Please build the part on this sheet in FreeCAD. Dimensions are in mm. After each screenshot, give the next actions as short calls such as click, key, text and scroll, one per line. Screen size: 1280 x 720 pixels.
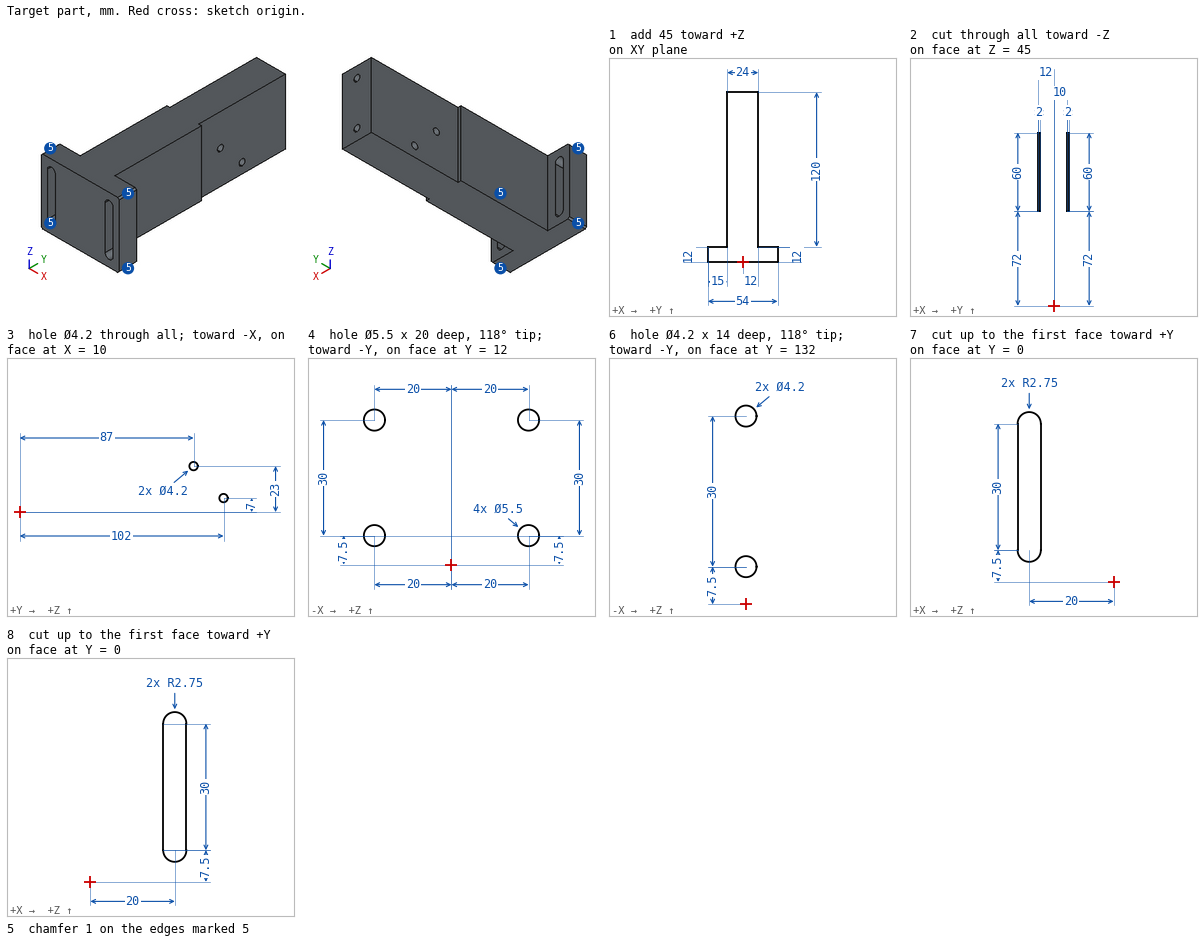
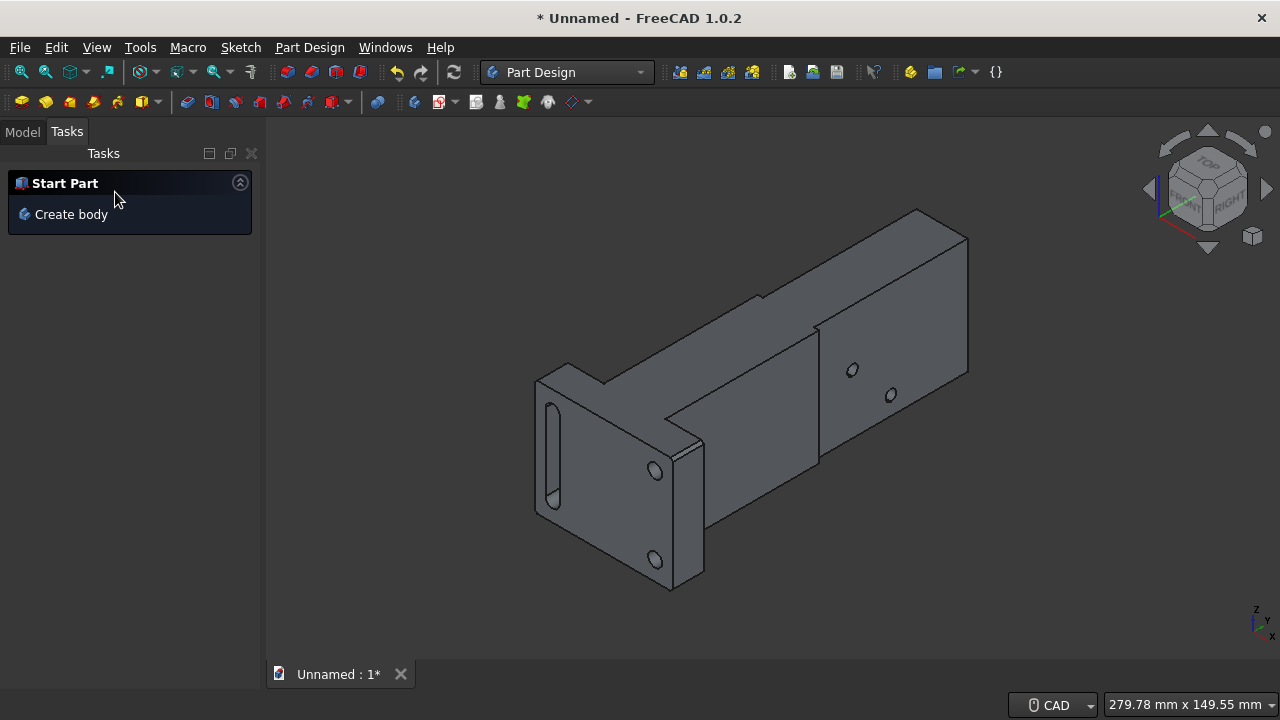
click(604, 485)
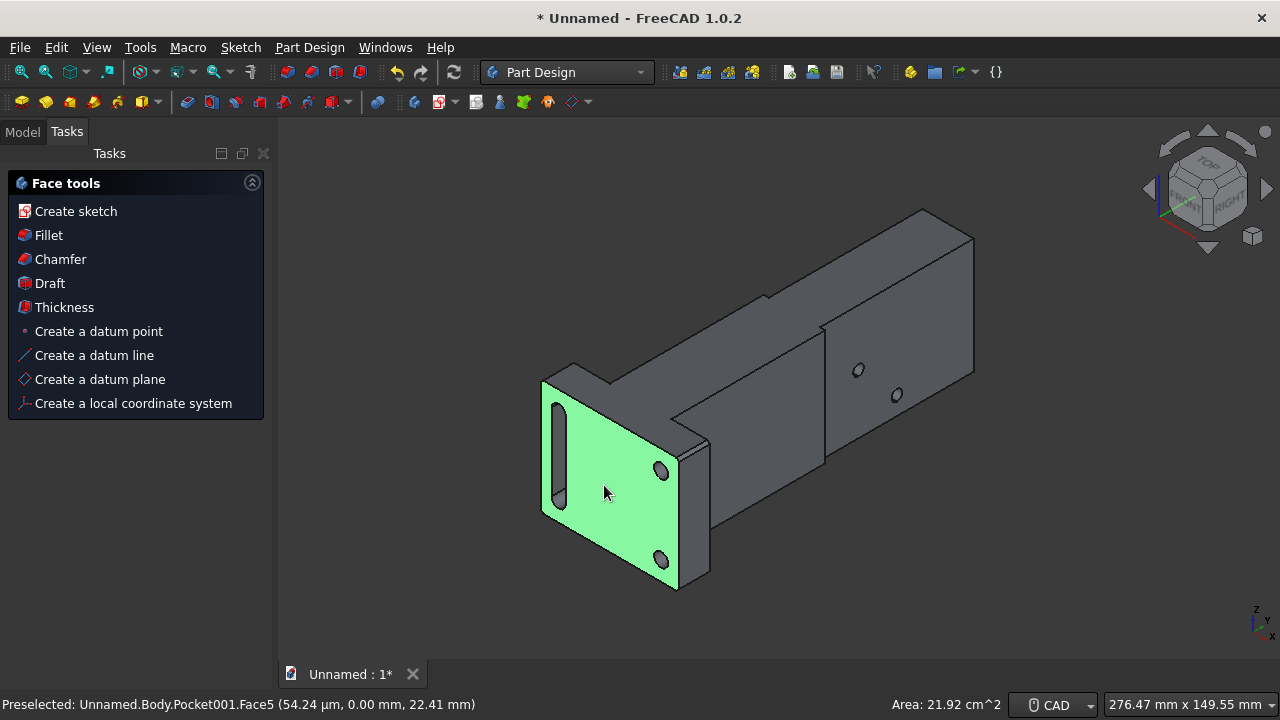
click(440, 102)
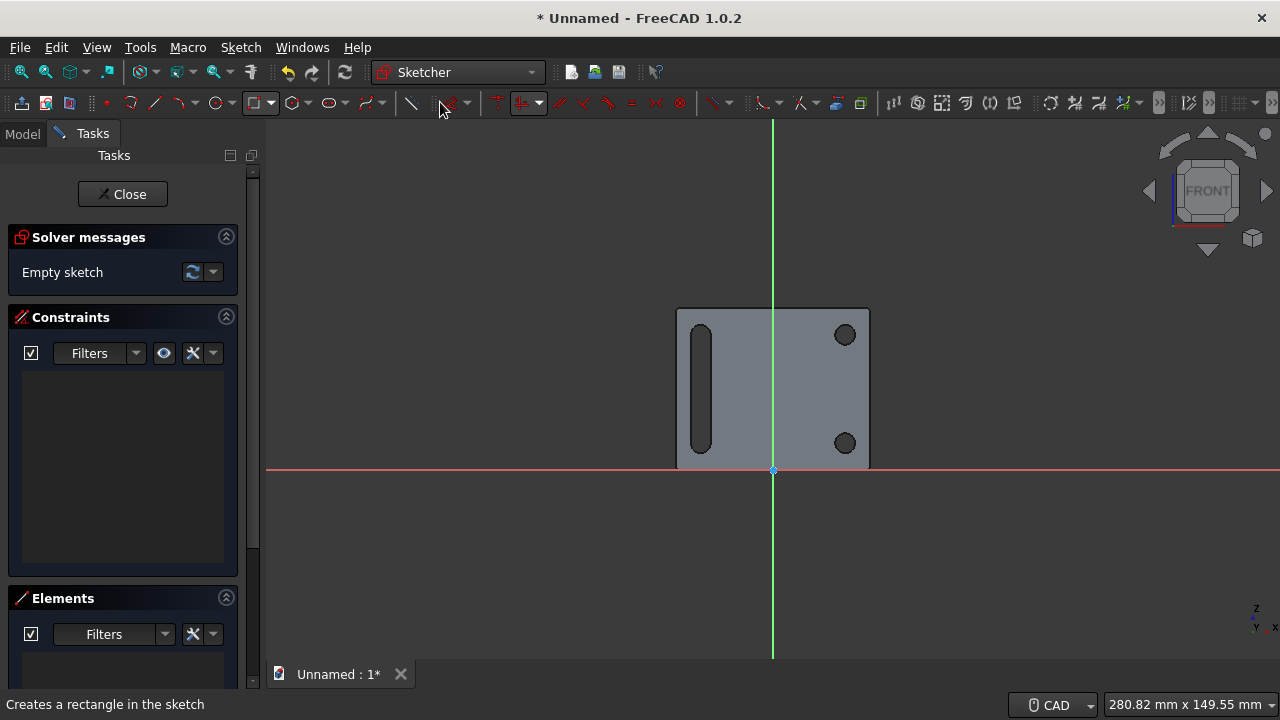
scroll(903, 405, up, 4)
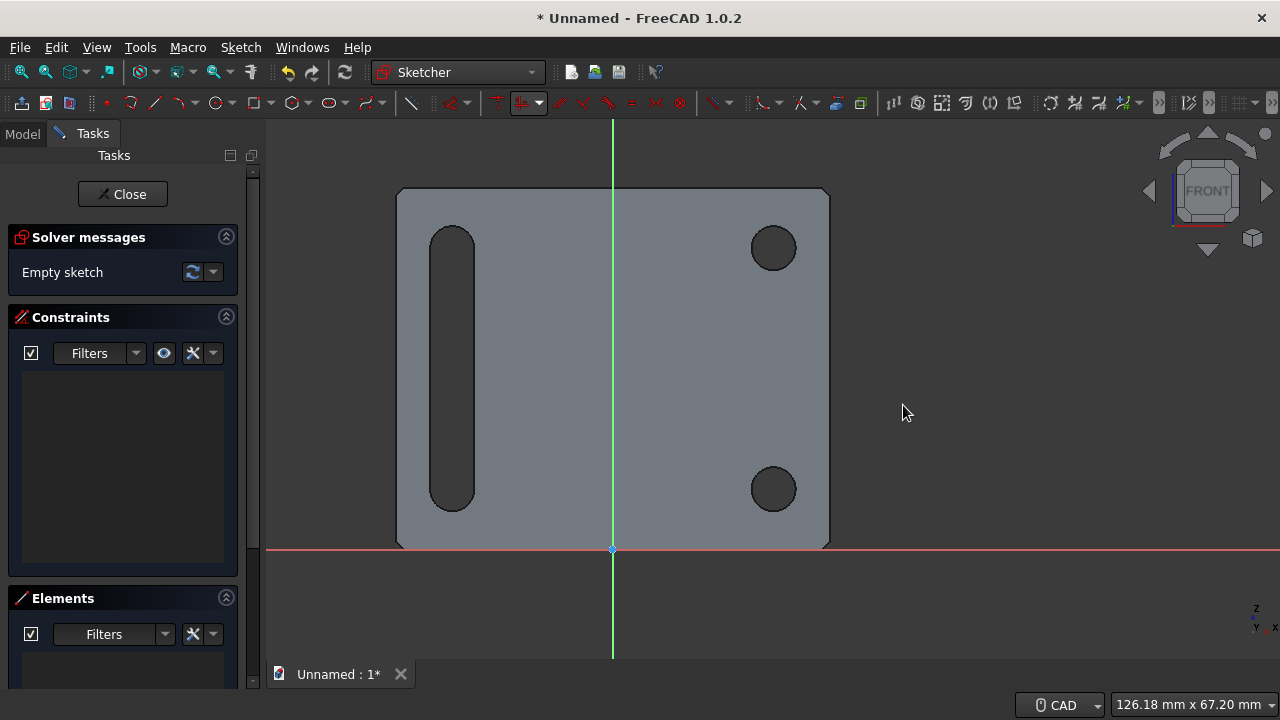
click(330, 104)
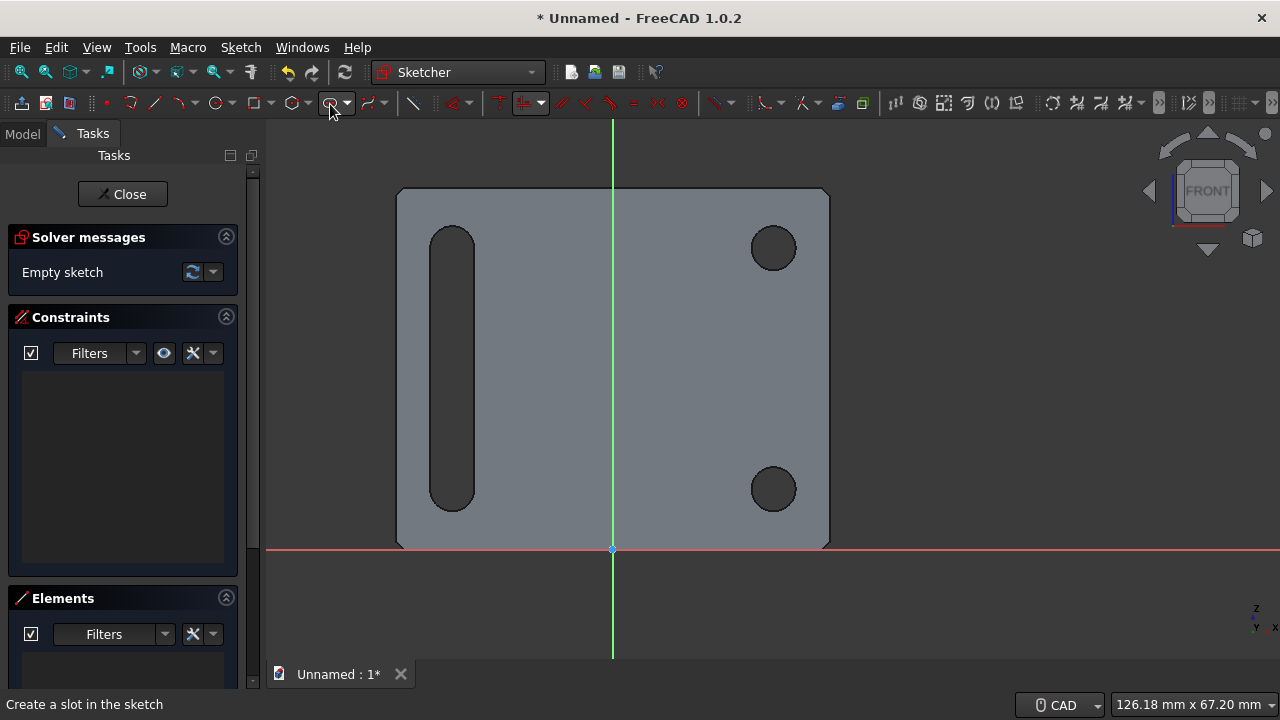
click(774, 489)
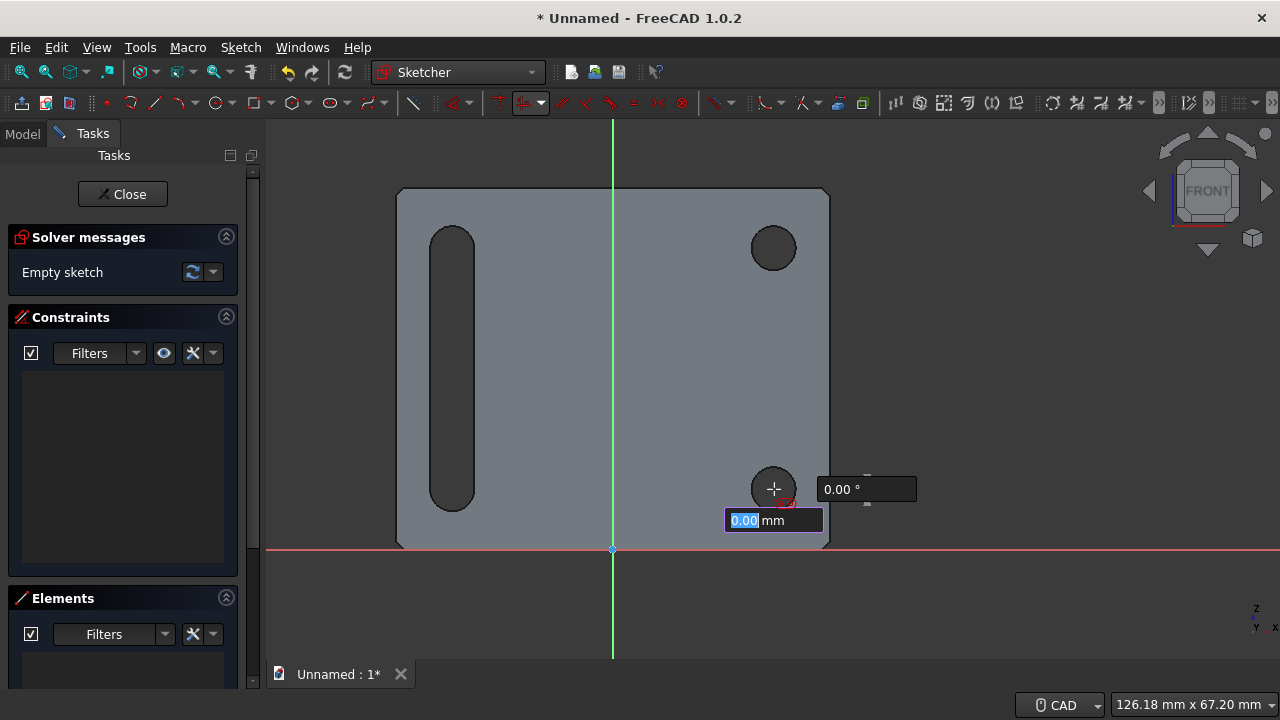
click(774, 248)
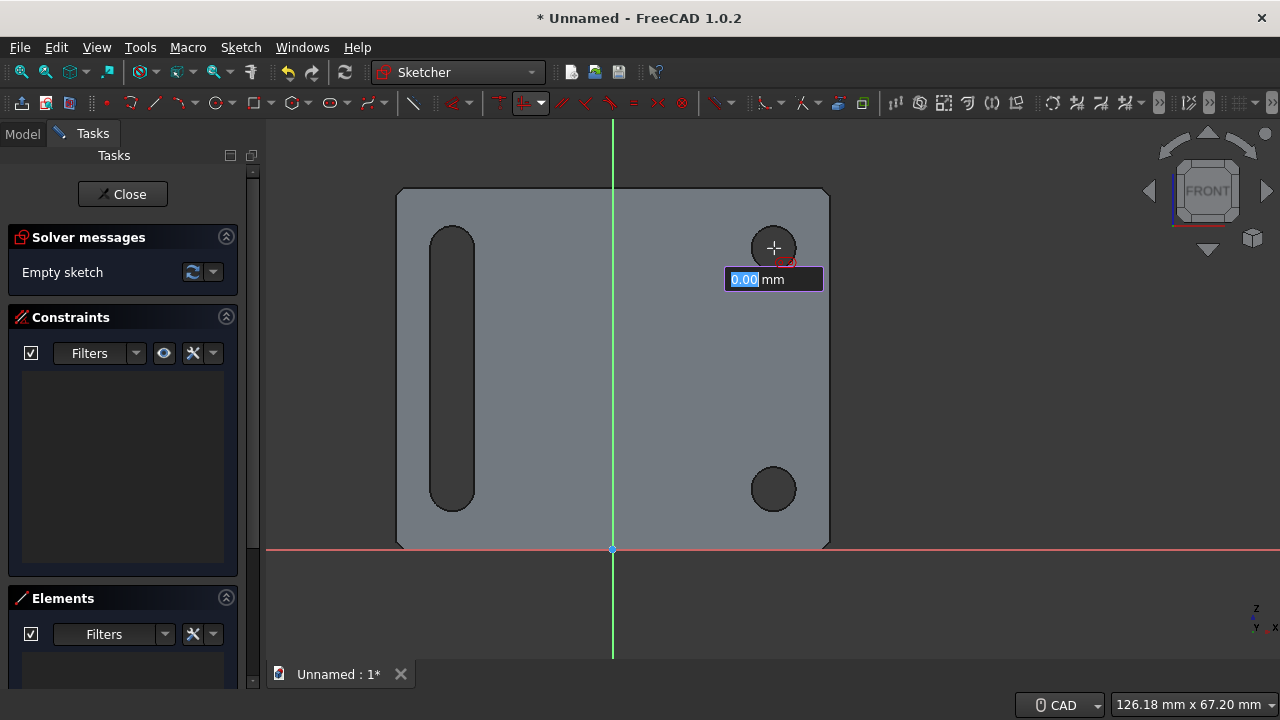
click(796, 369)
key(Escape)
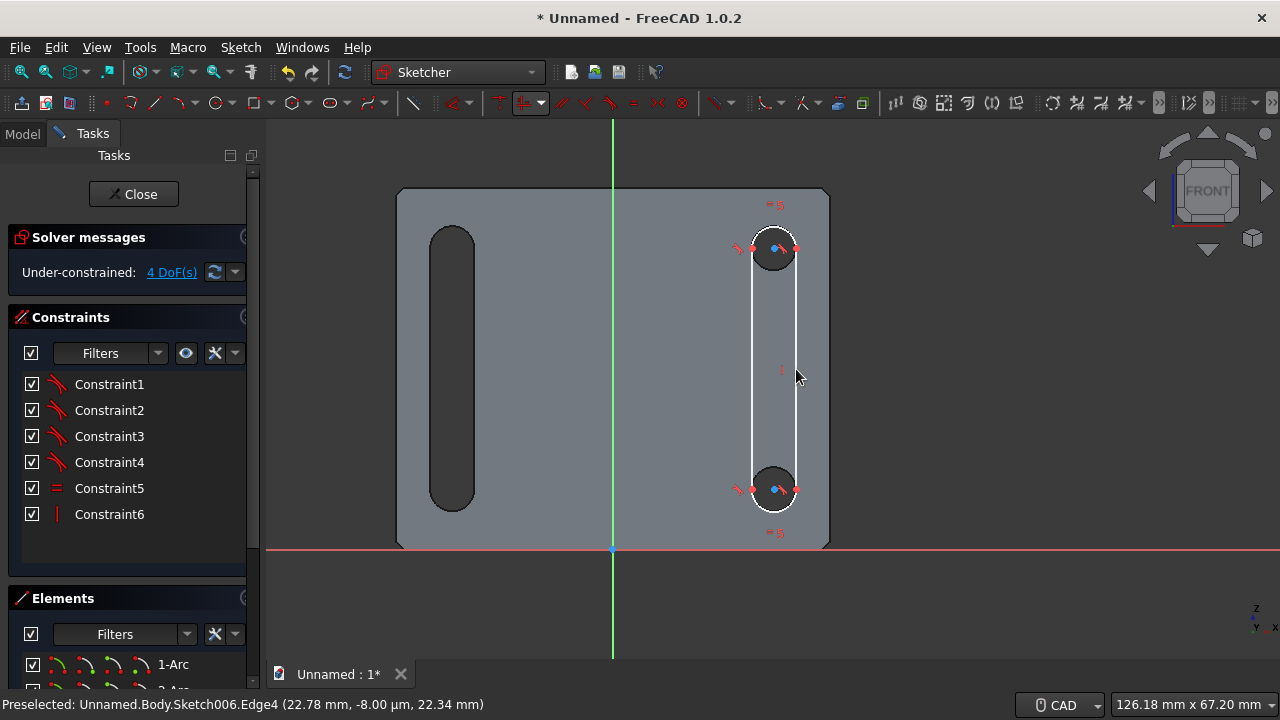
click(452, 104)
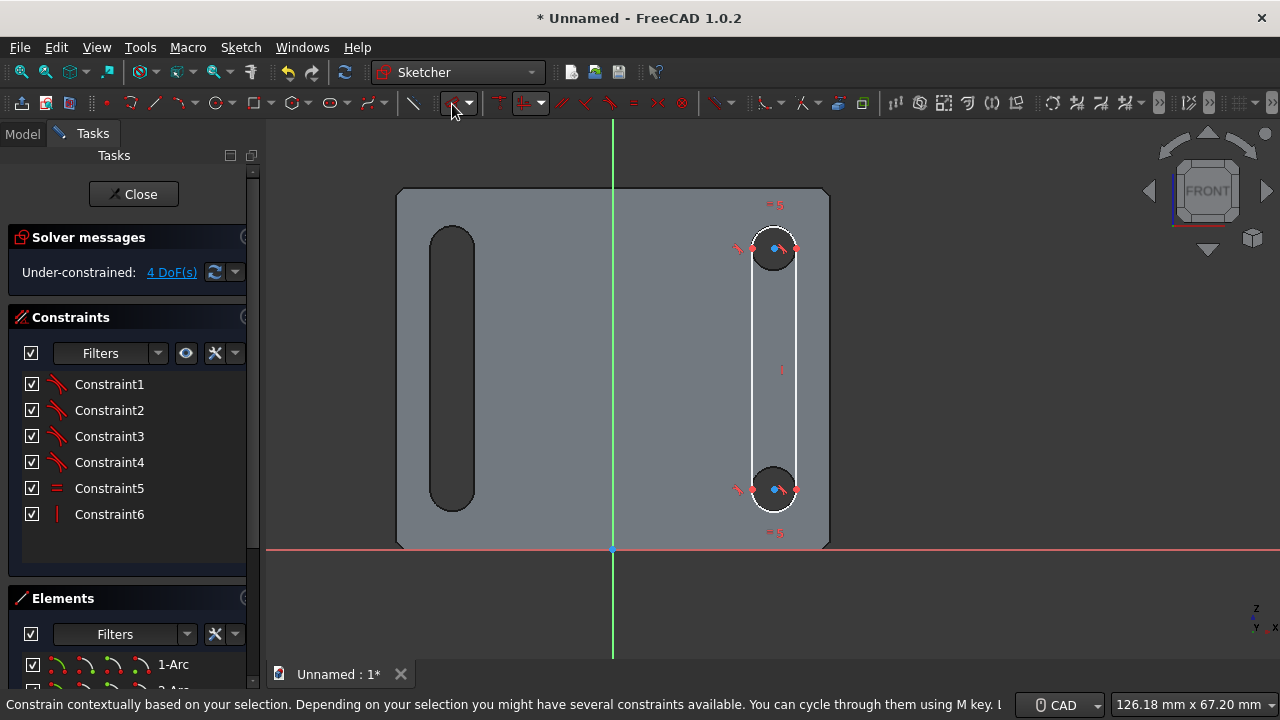
scroll(761, 508, up, 3)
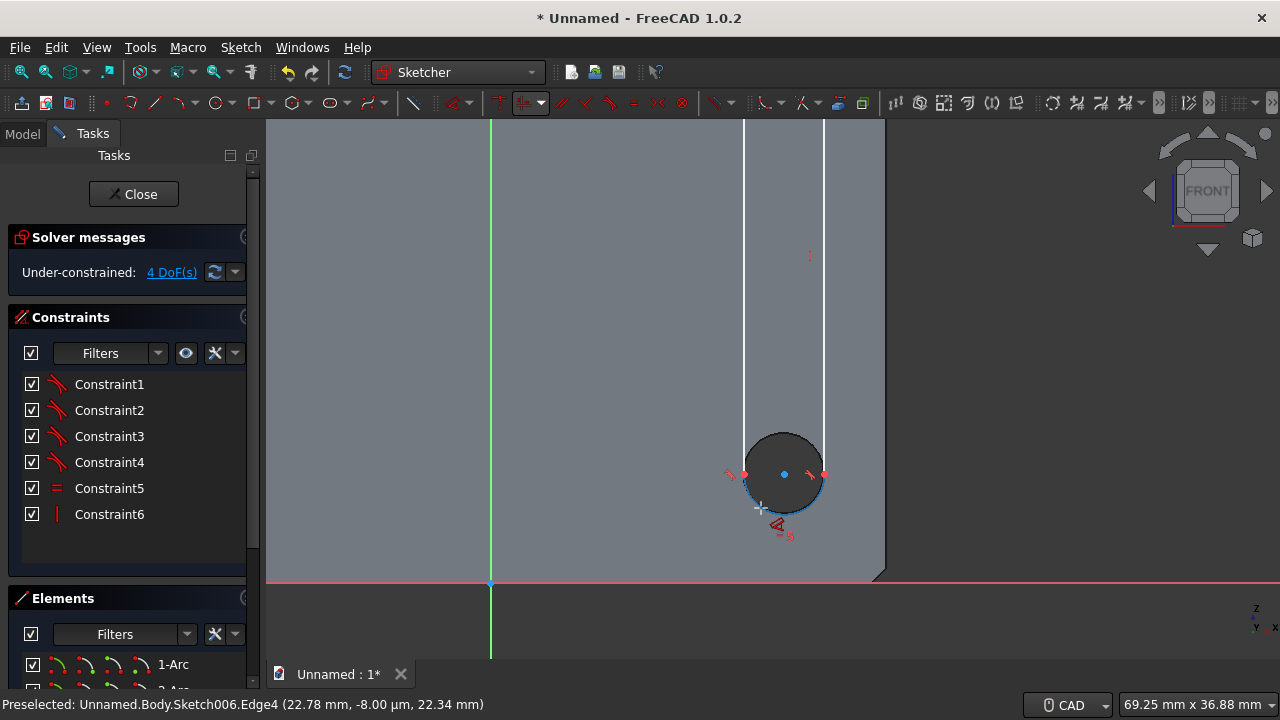
click(761, 507)
click(742, 533)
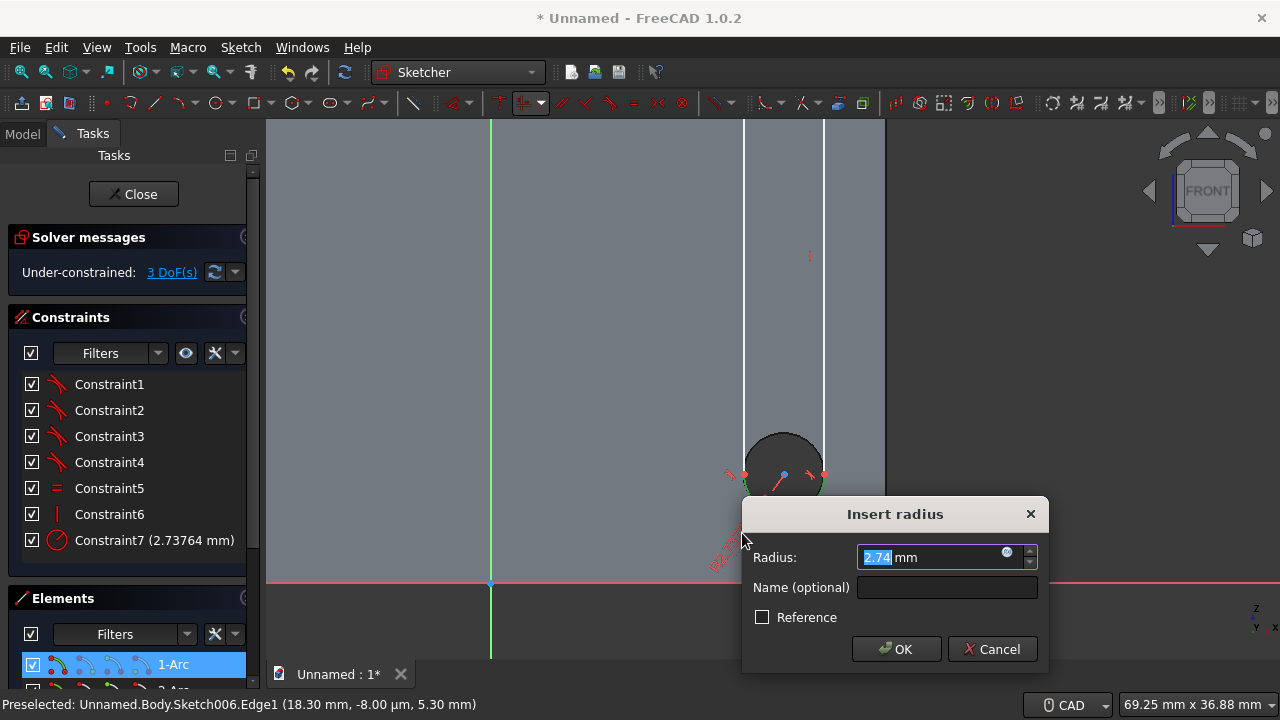
text(2.75)
key(Return)